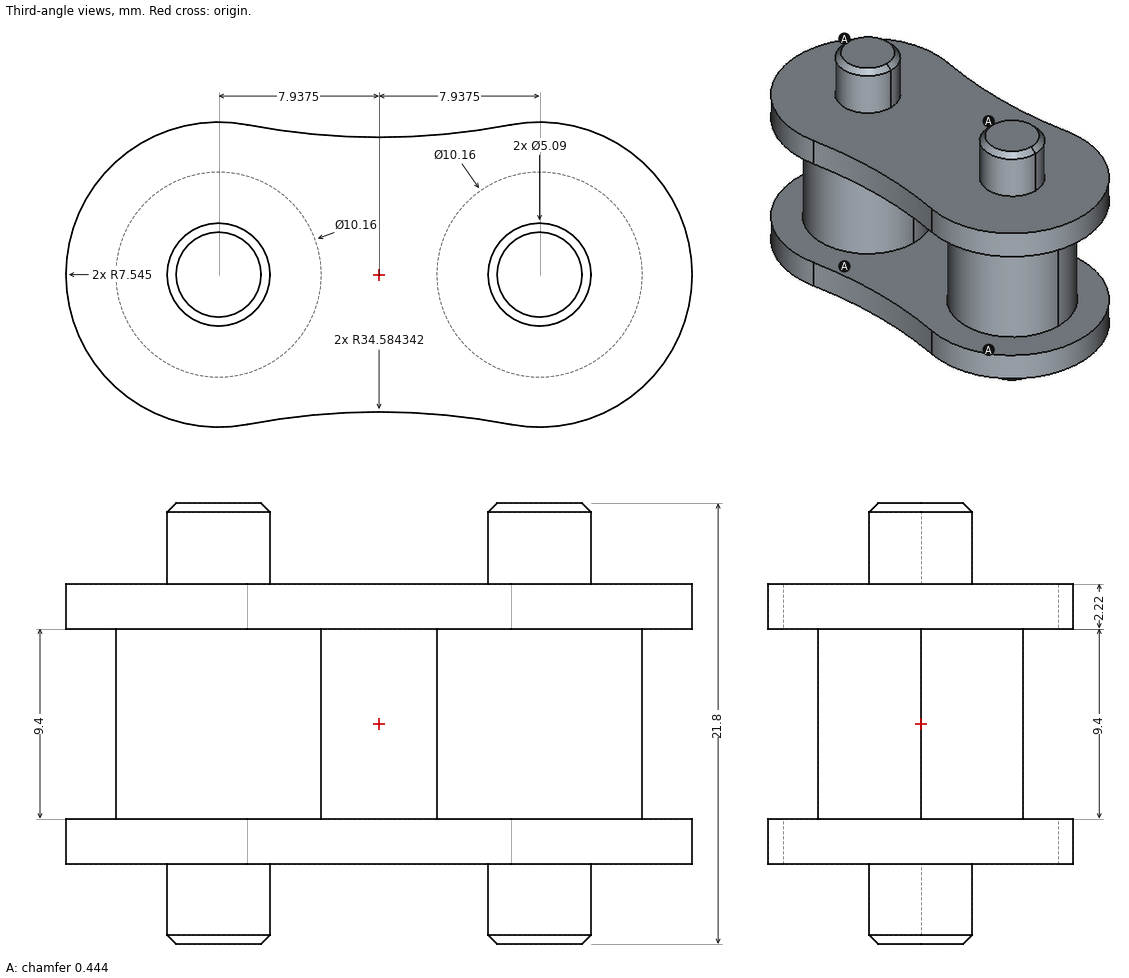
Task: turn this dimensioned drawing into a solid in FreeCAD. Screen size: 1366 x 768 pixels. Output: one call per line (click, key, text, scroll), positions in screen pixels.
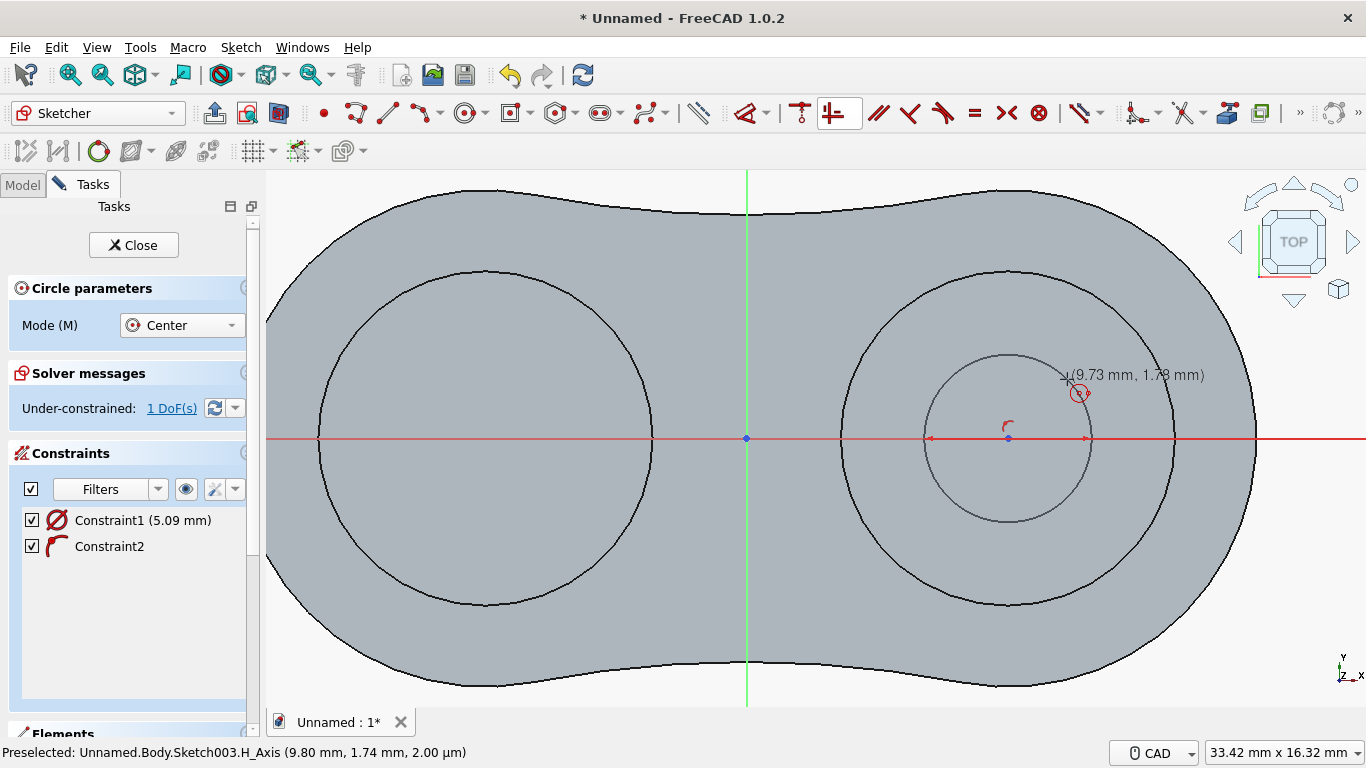
click(485, 438)
move(545, 379)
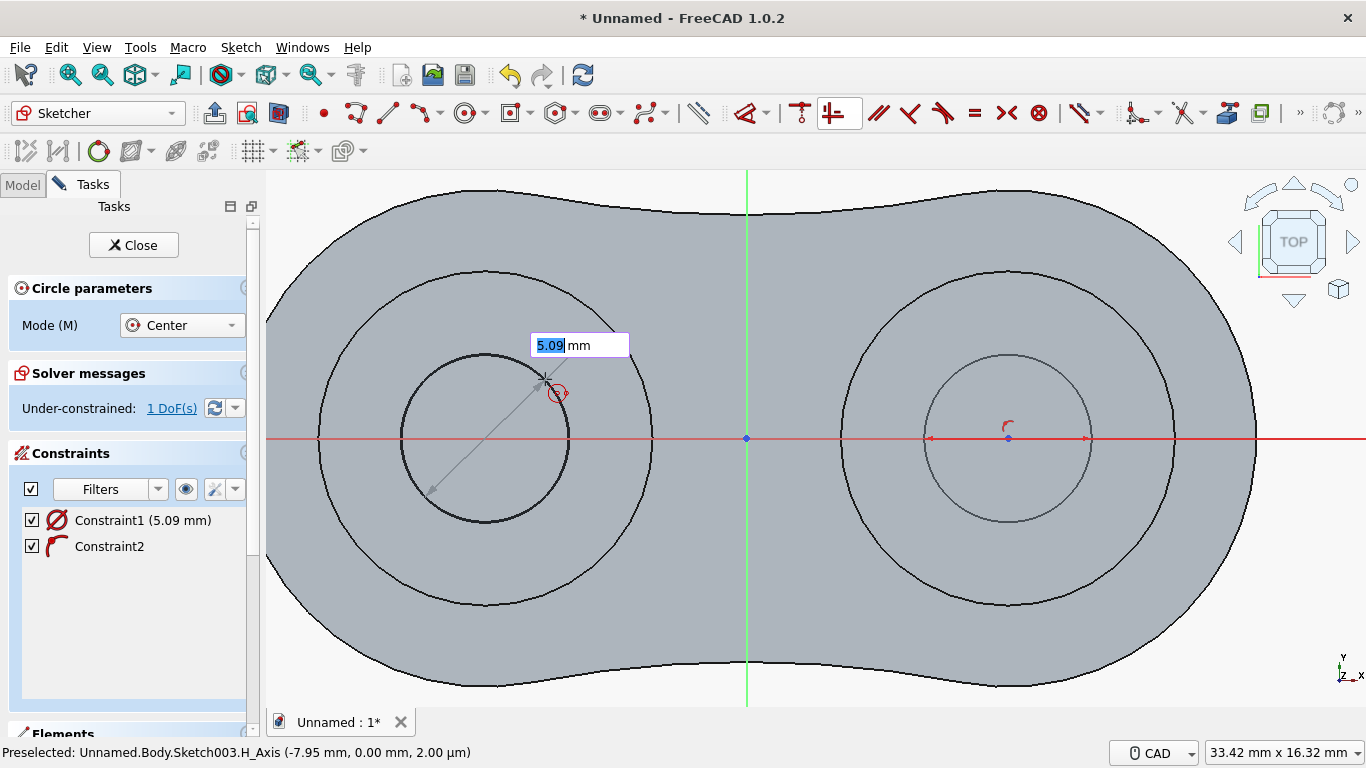
text(5.09)
key(Return)
key(Escape)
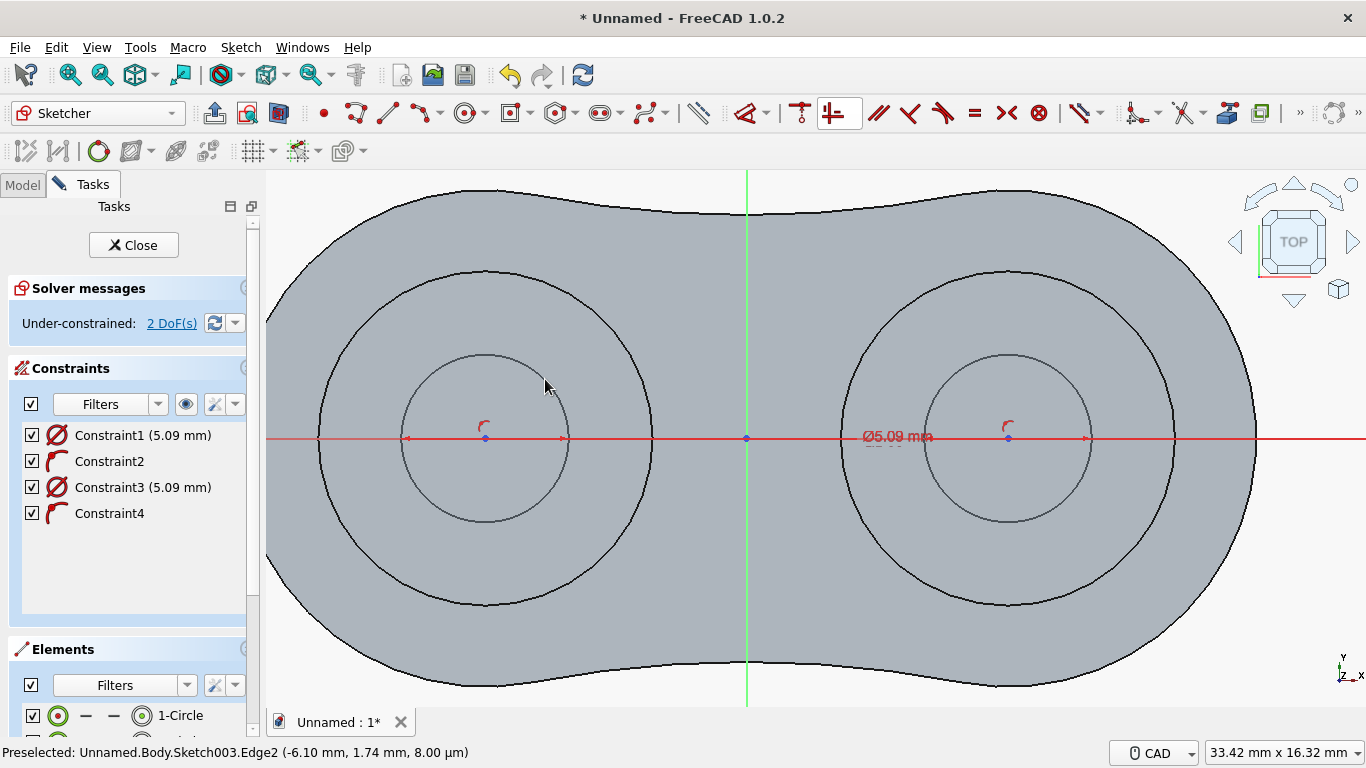
key(d)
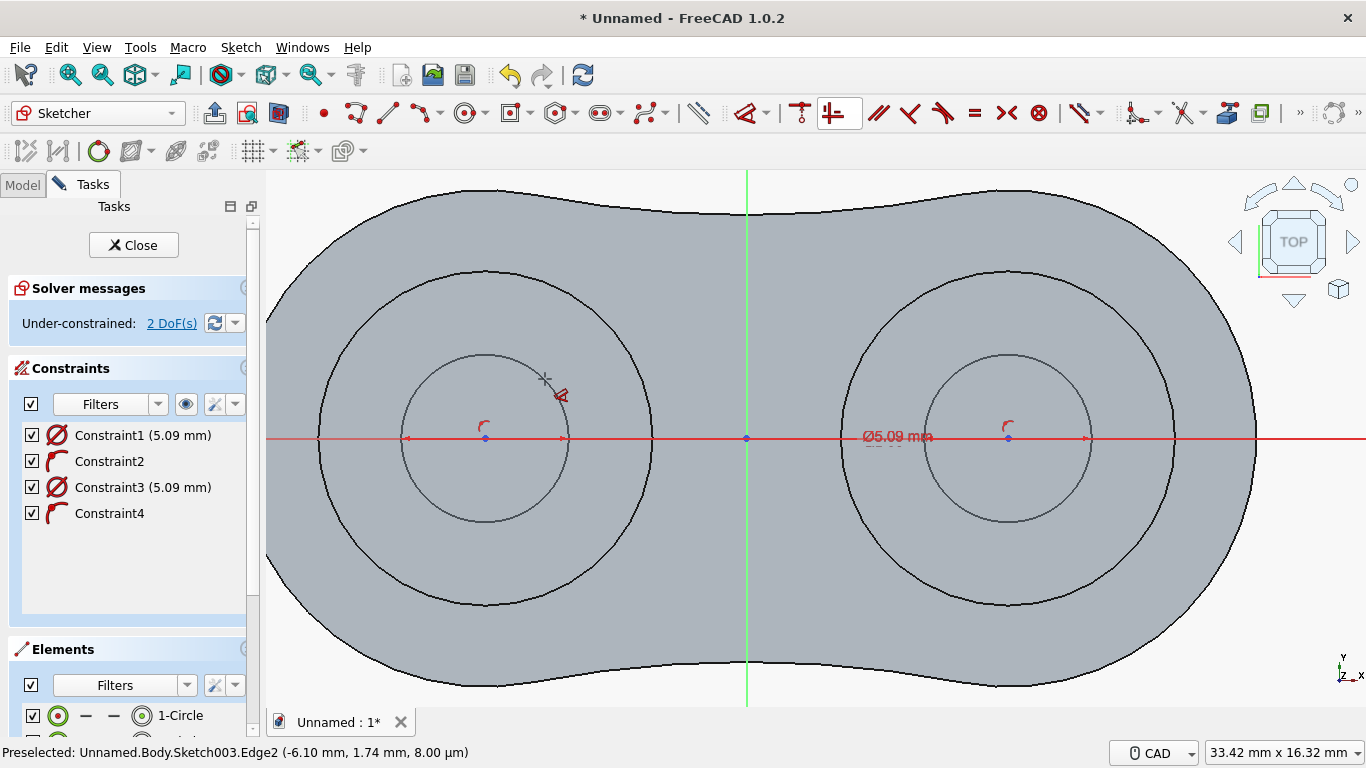
click(1008, 438)
click(877, 472)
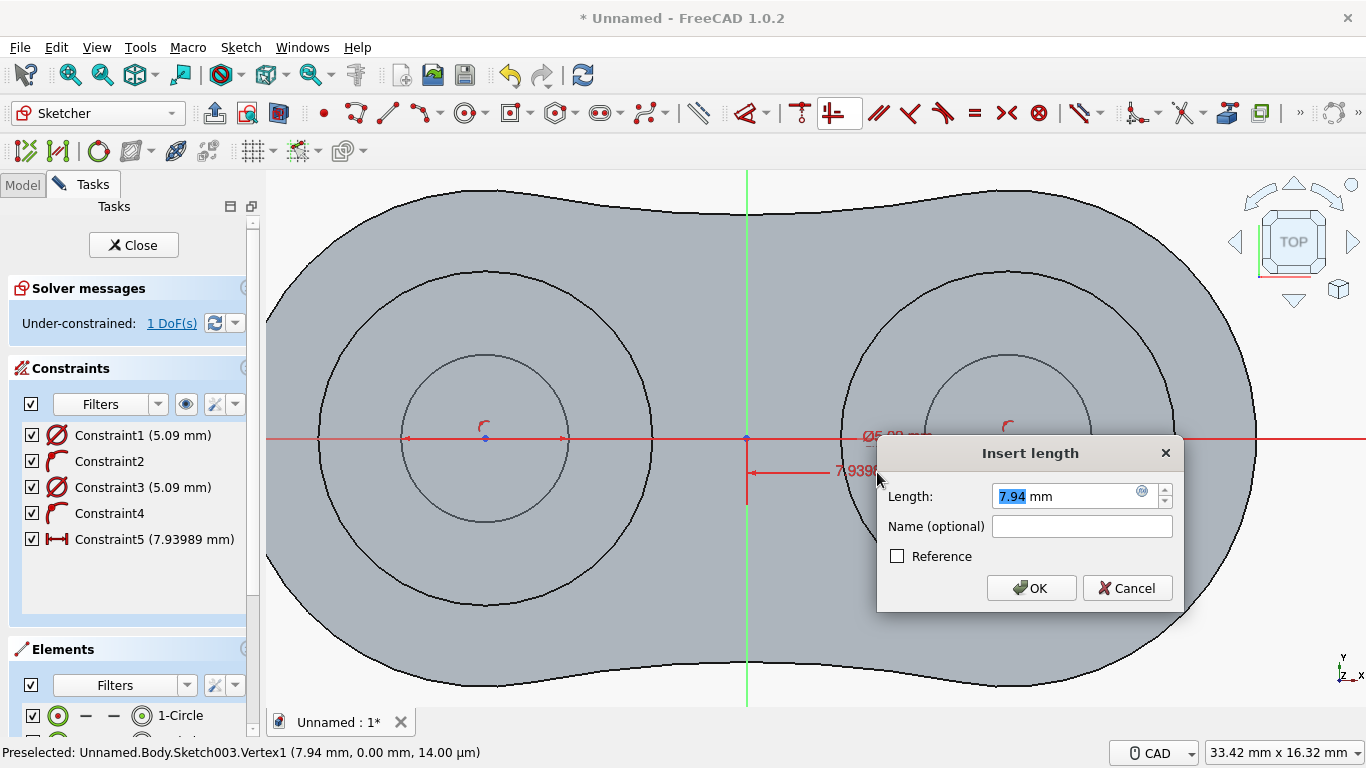
text(7.9375)
key(Return)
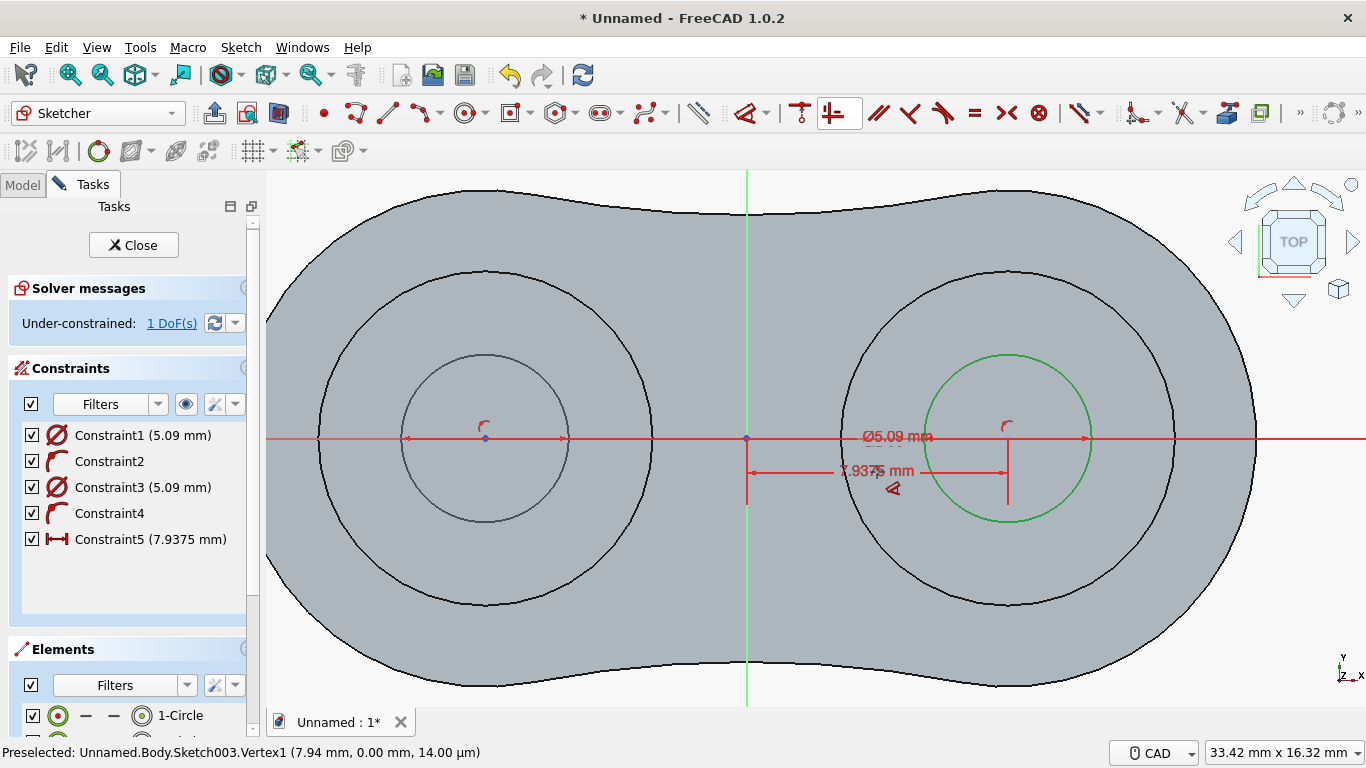
click(485, 438)
click(616, 472)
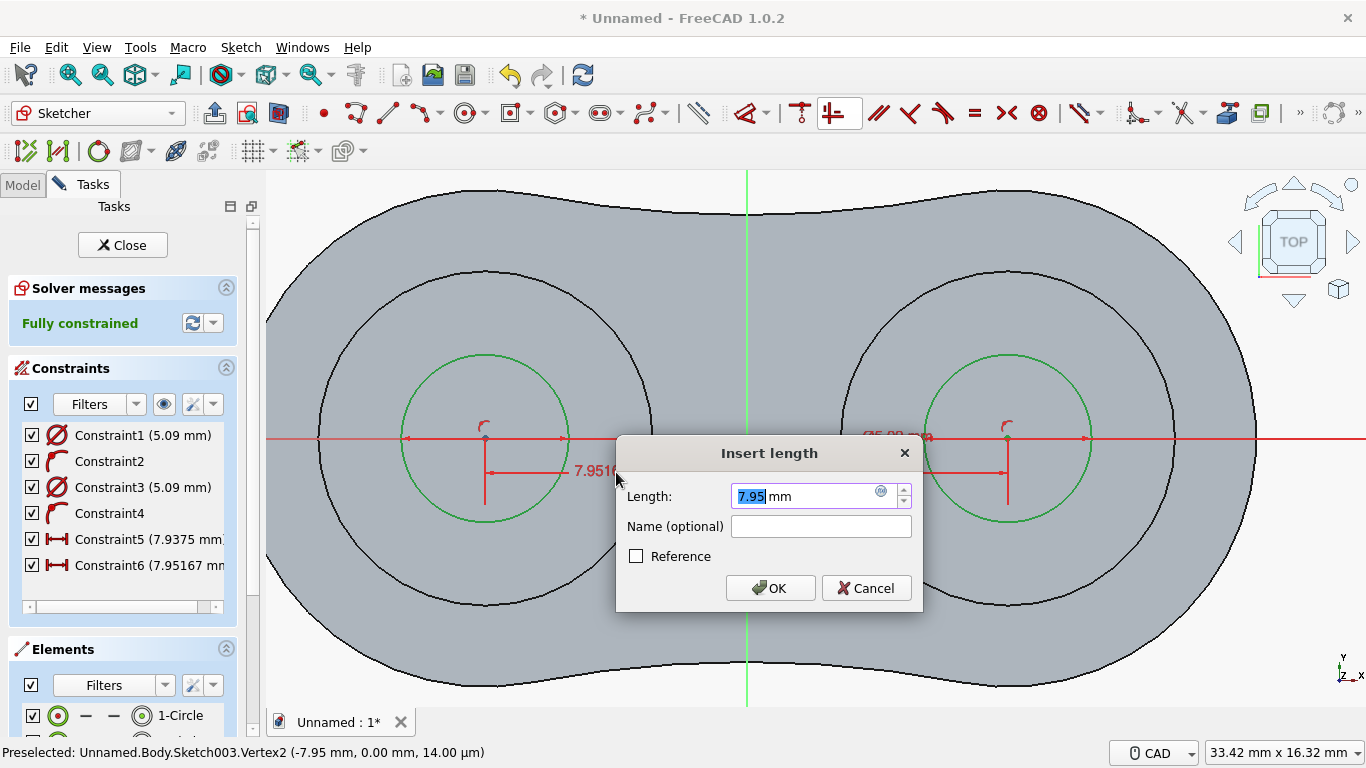
text(7.9375)
key(Return)
key(Escape)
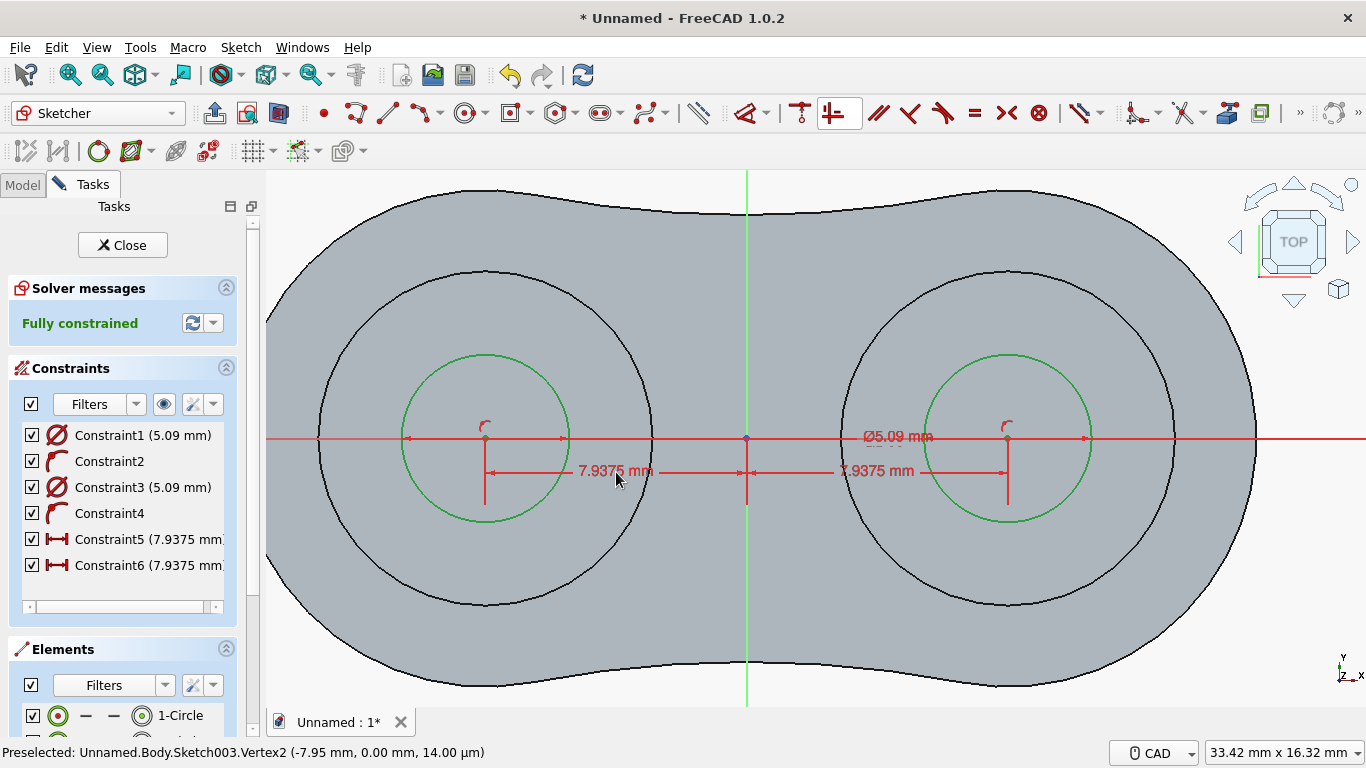
click(123, 245)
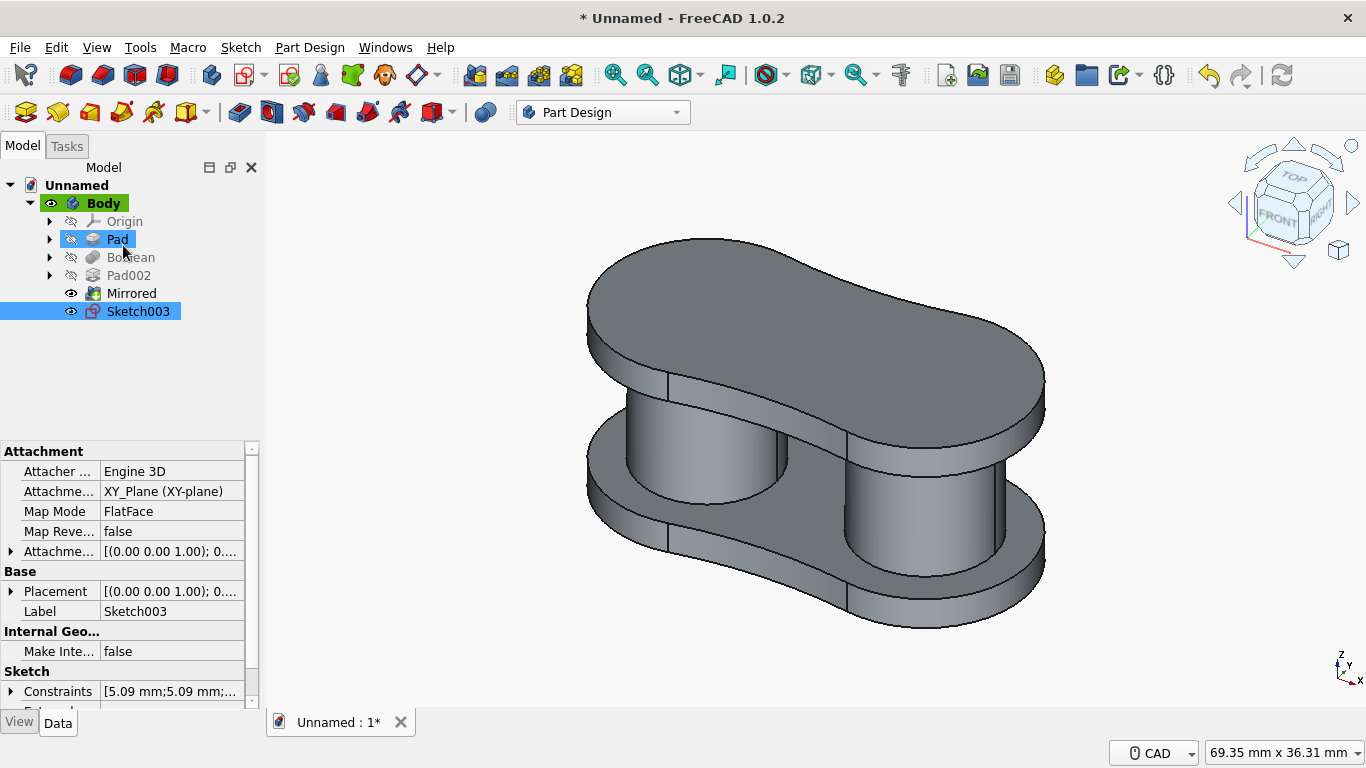
click(26, 112)